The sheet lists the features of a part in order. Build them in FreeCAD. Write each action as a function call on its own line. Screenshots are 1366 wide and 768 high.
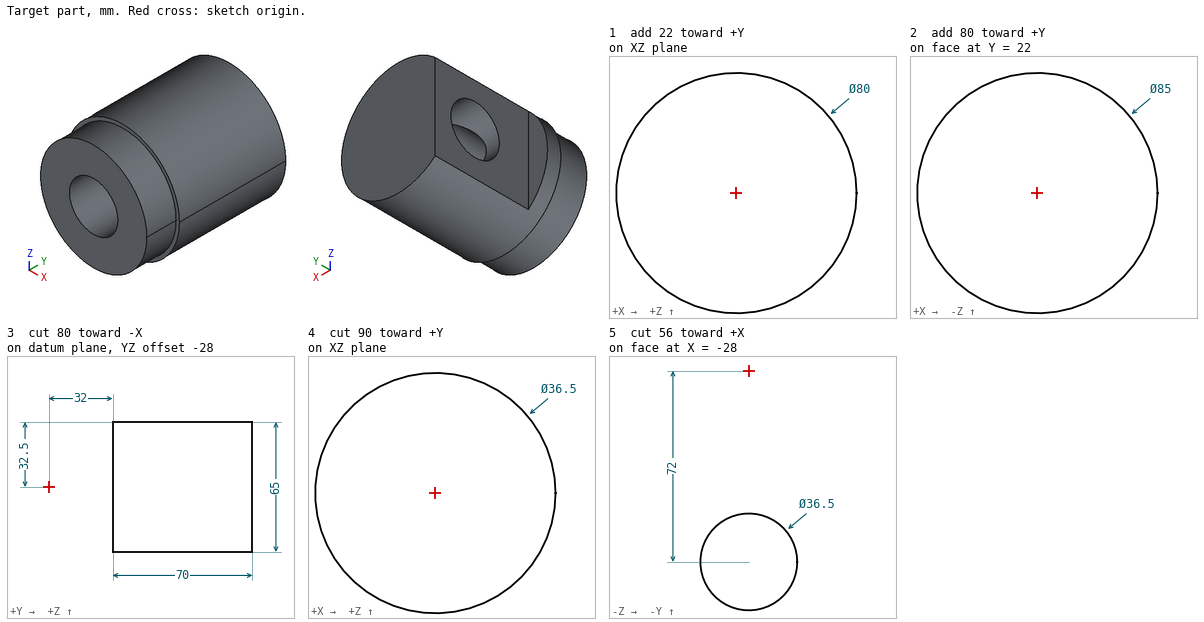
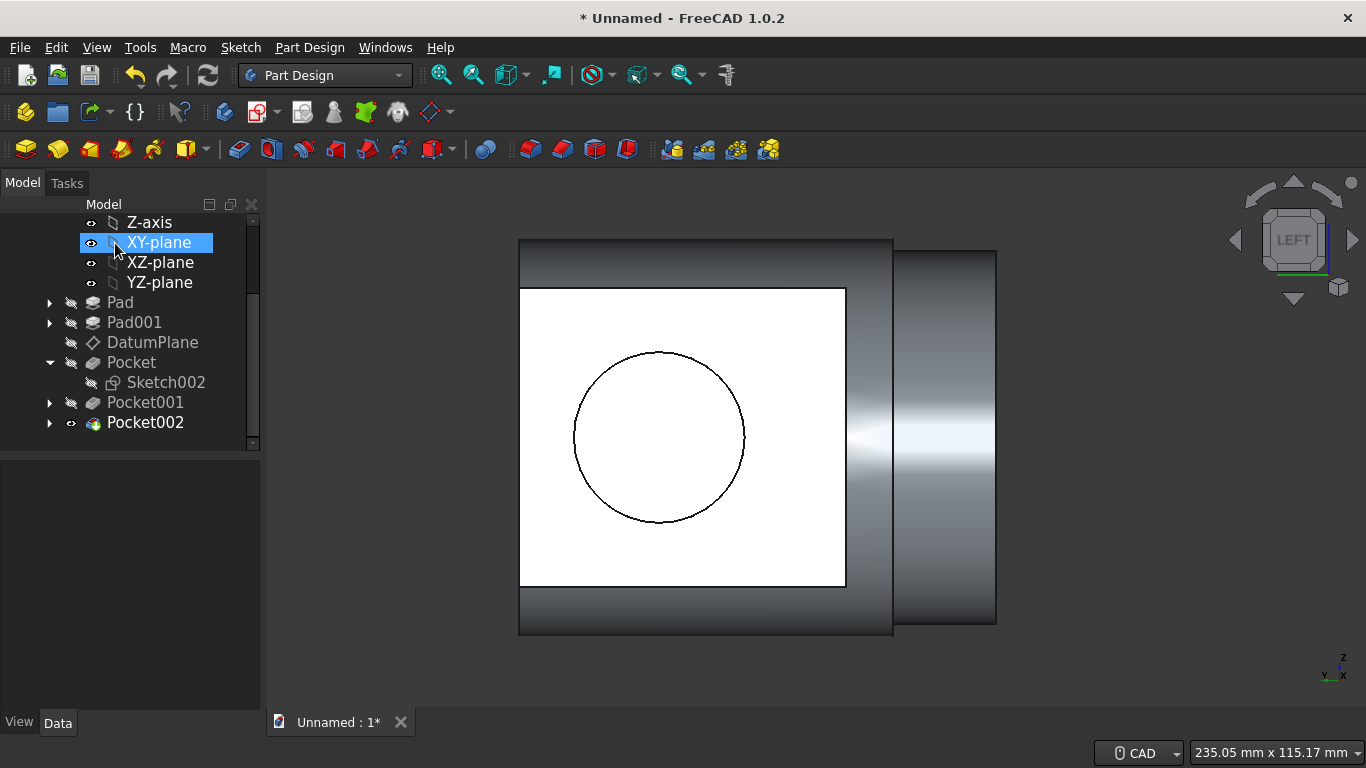
key(0)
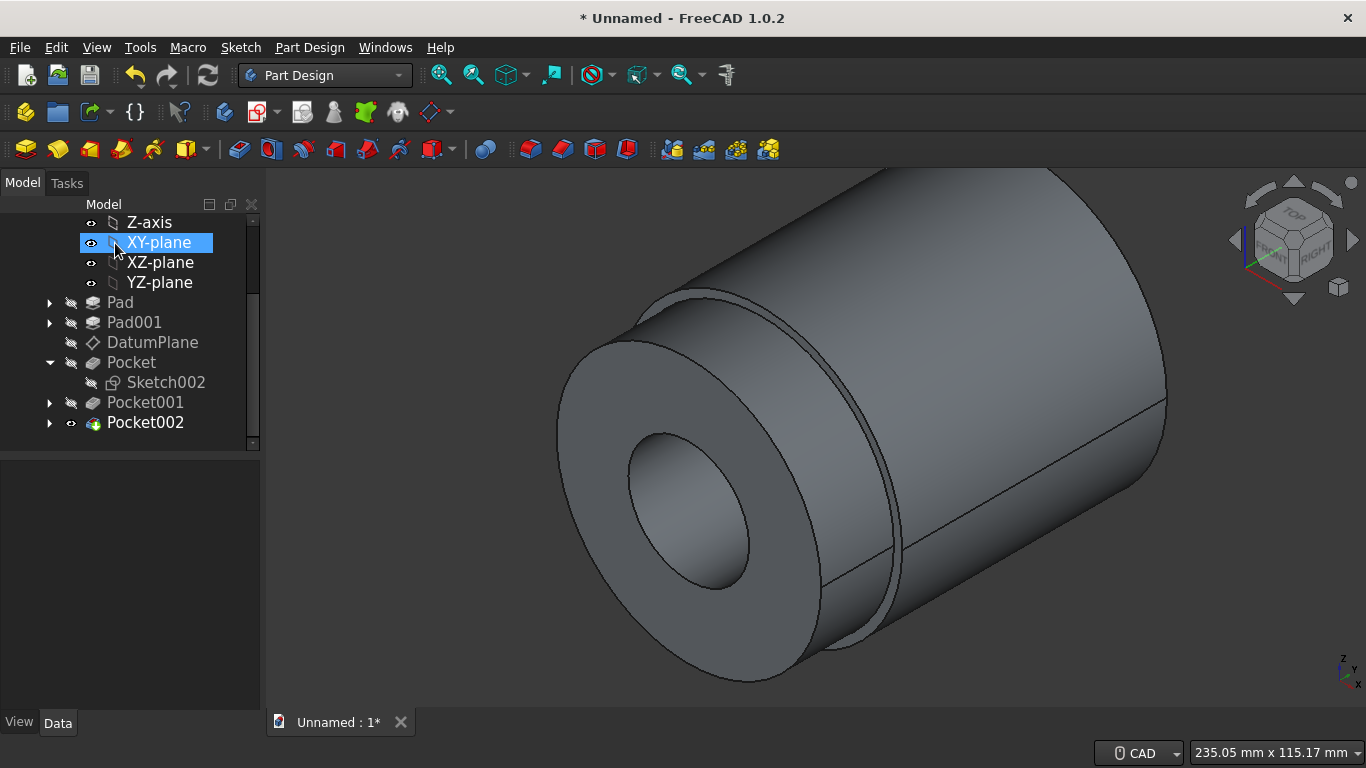
click(442, 76)